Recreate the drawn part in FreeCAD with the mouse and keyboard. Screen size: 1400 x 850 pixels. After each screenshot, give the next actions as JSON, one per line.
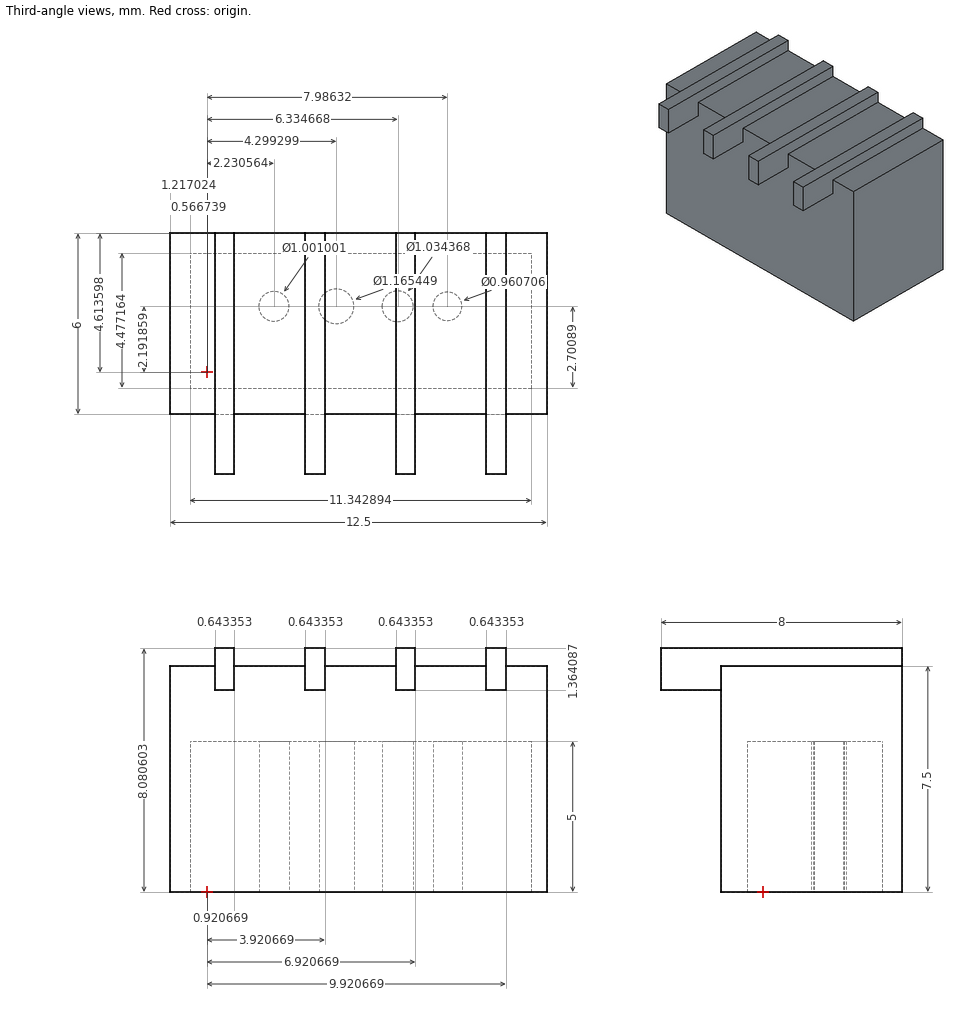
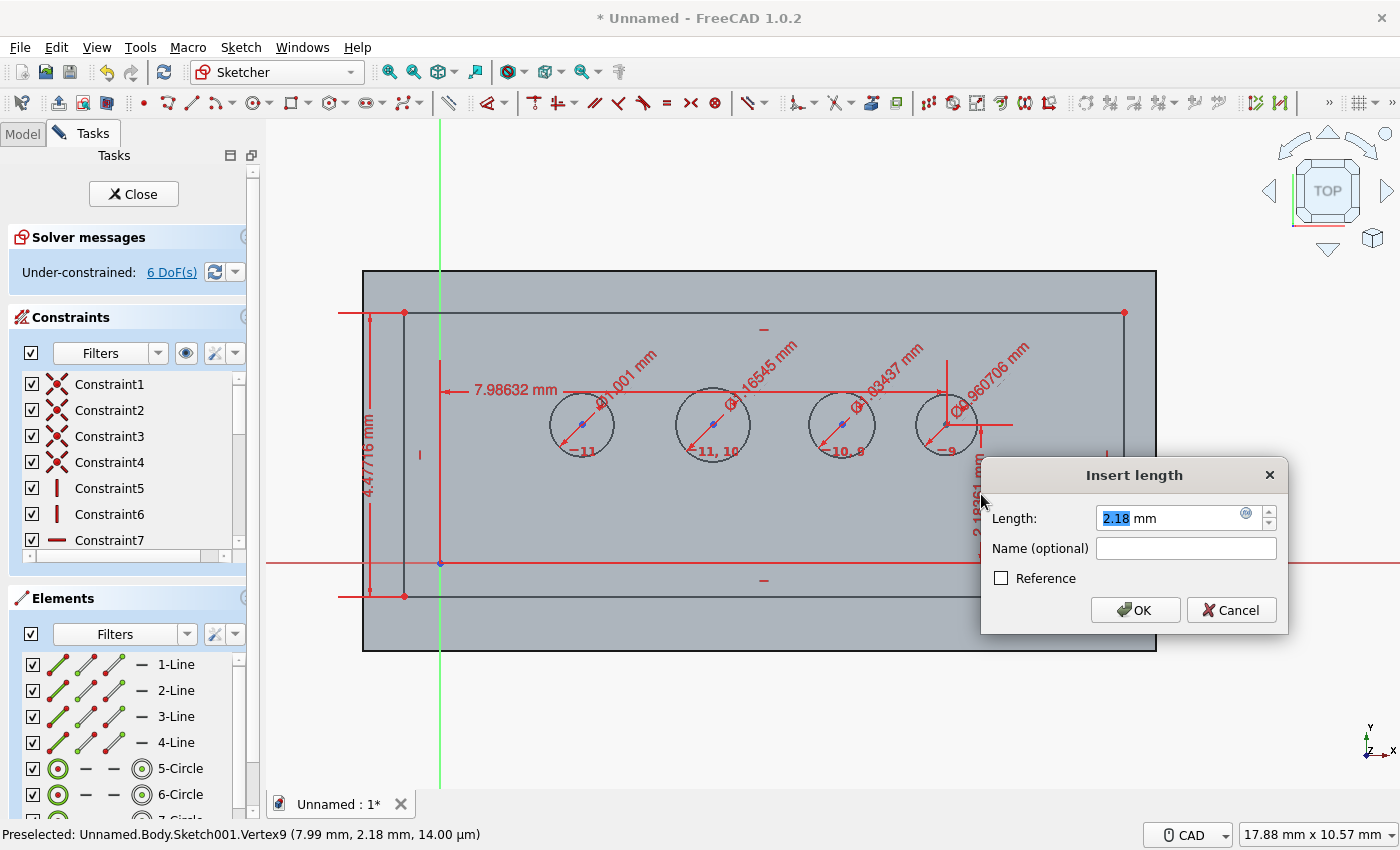
{"action": "type", "text": "2.191859"}
{"action": "key", "text": "Return"}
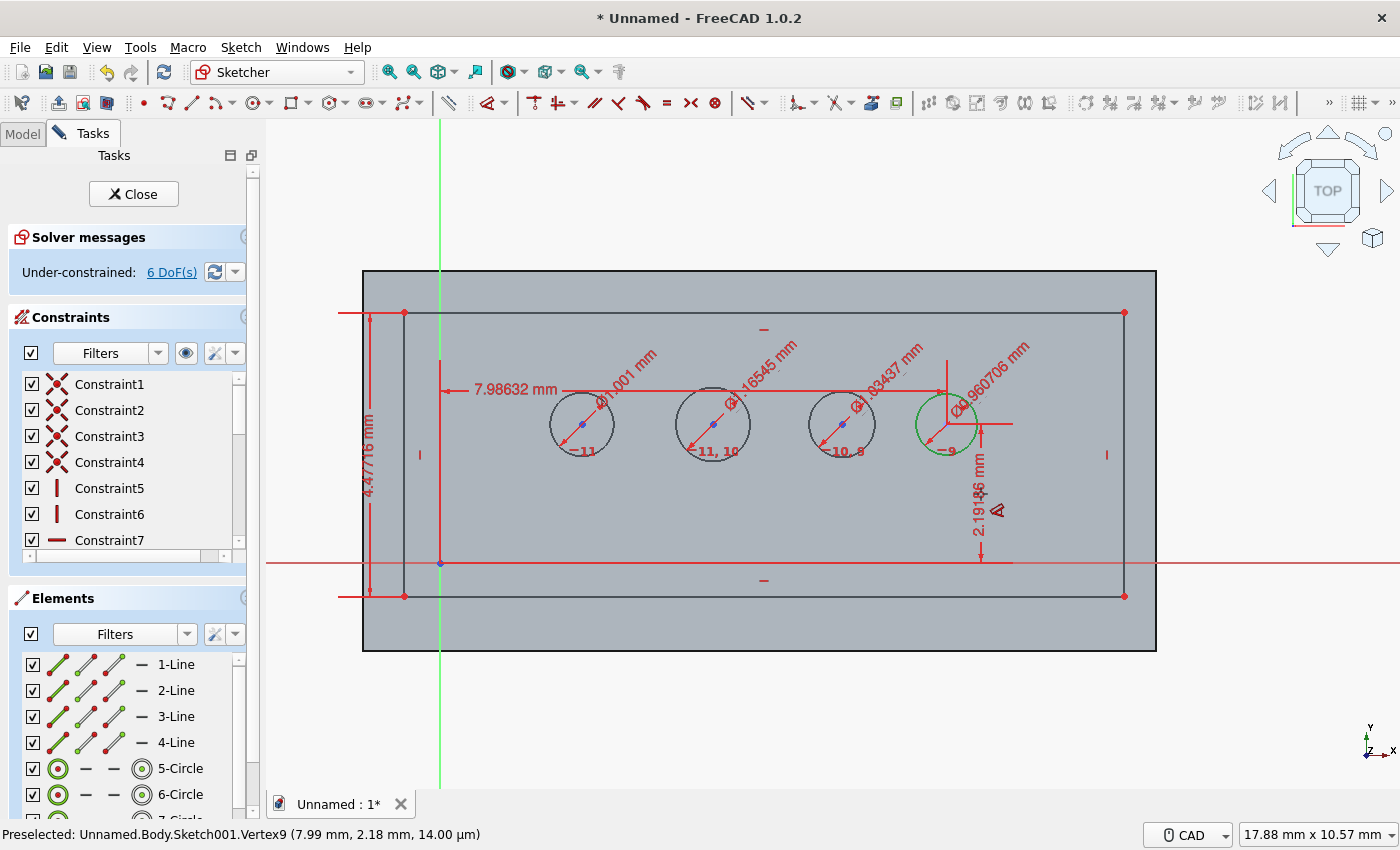
{"action": "left_click", "coordinate": [842, 424]}
{"action": "left_click", "coordinate": [641, 621]}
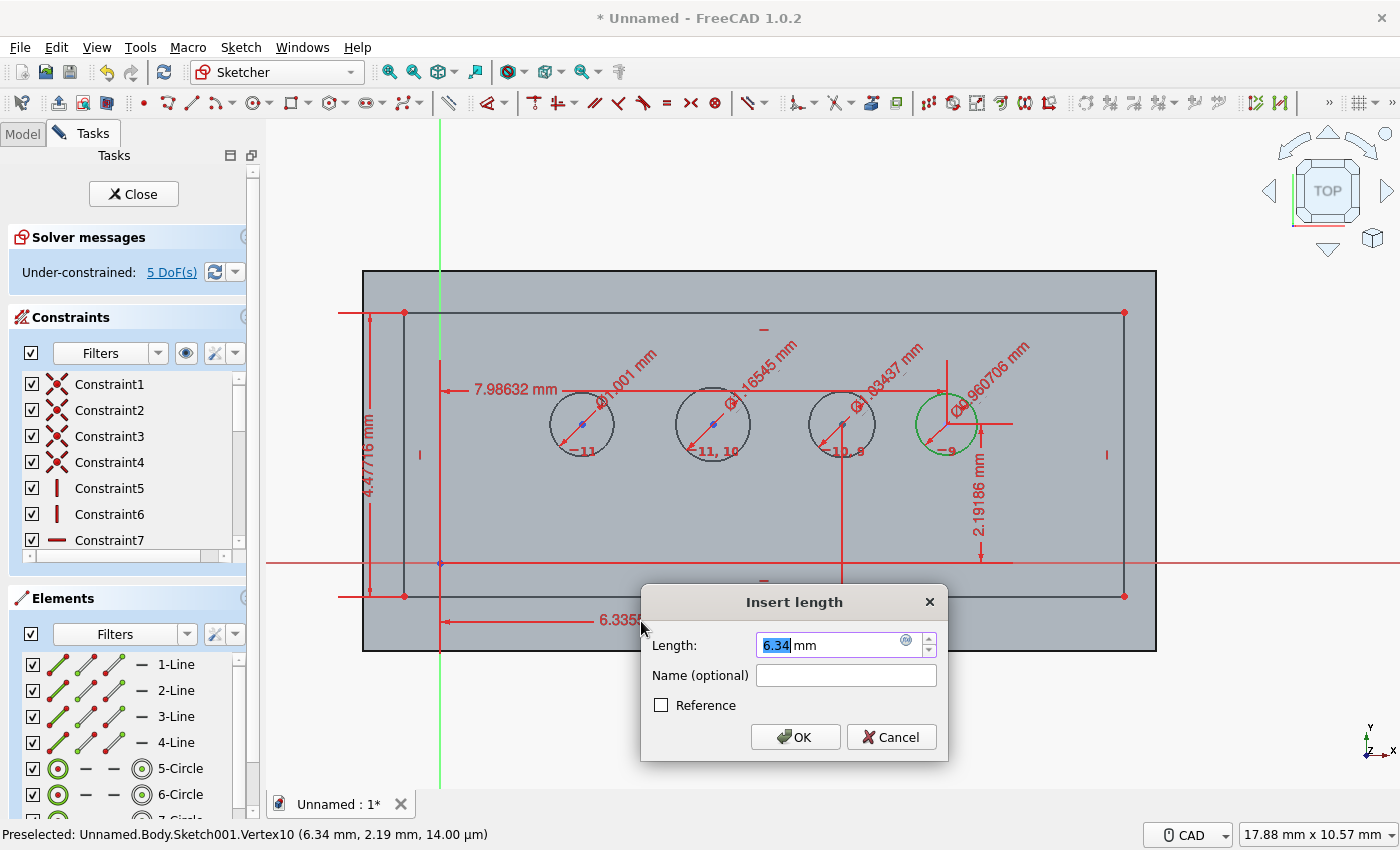
{"action": "type", "text": "6.334668"}
{"action": "key", "text": "Return"}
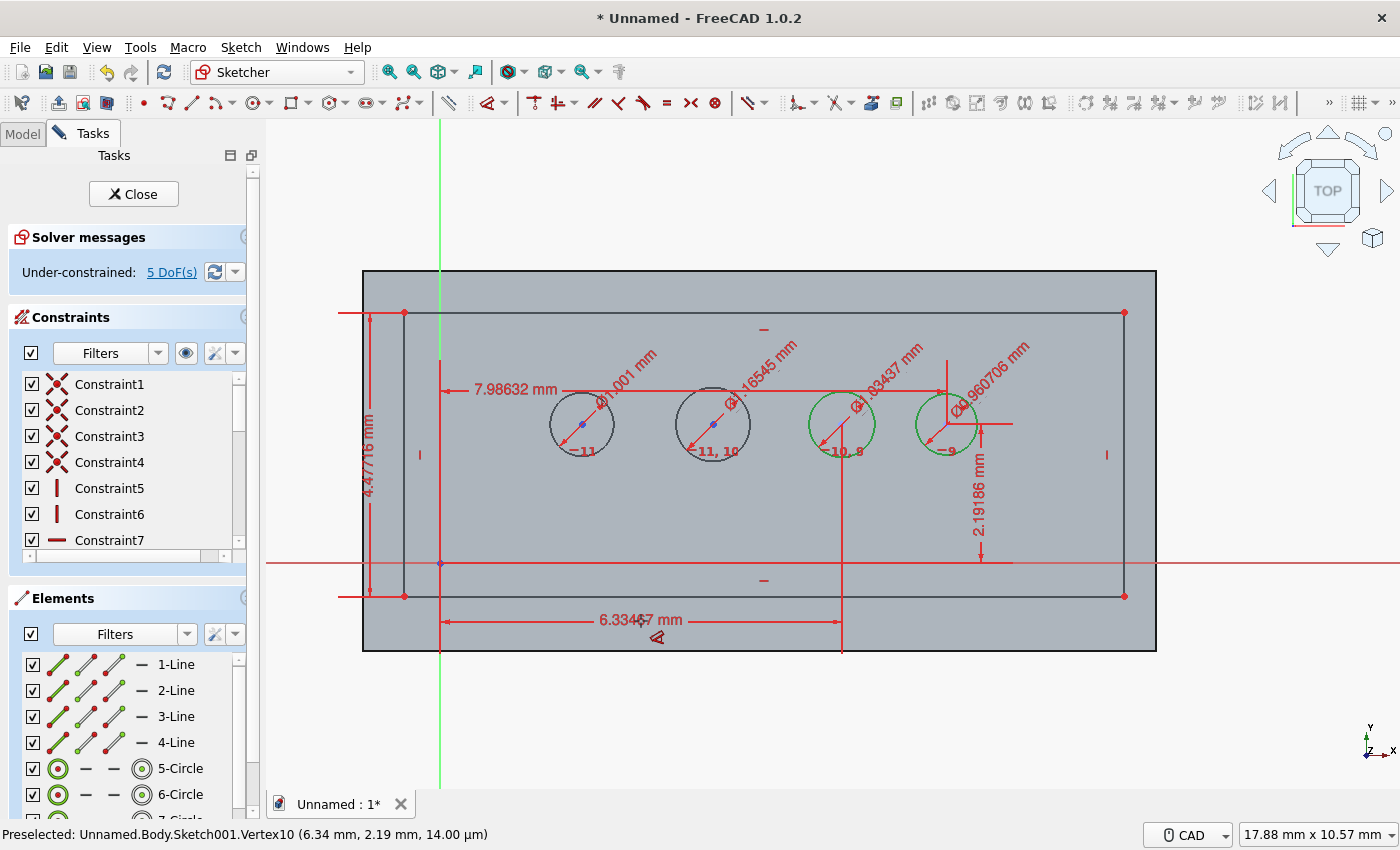
{"action": "left_click", "coordinate": [713, 424]}
{"action": "left_click", "coordinate": [514, 621]}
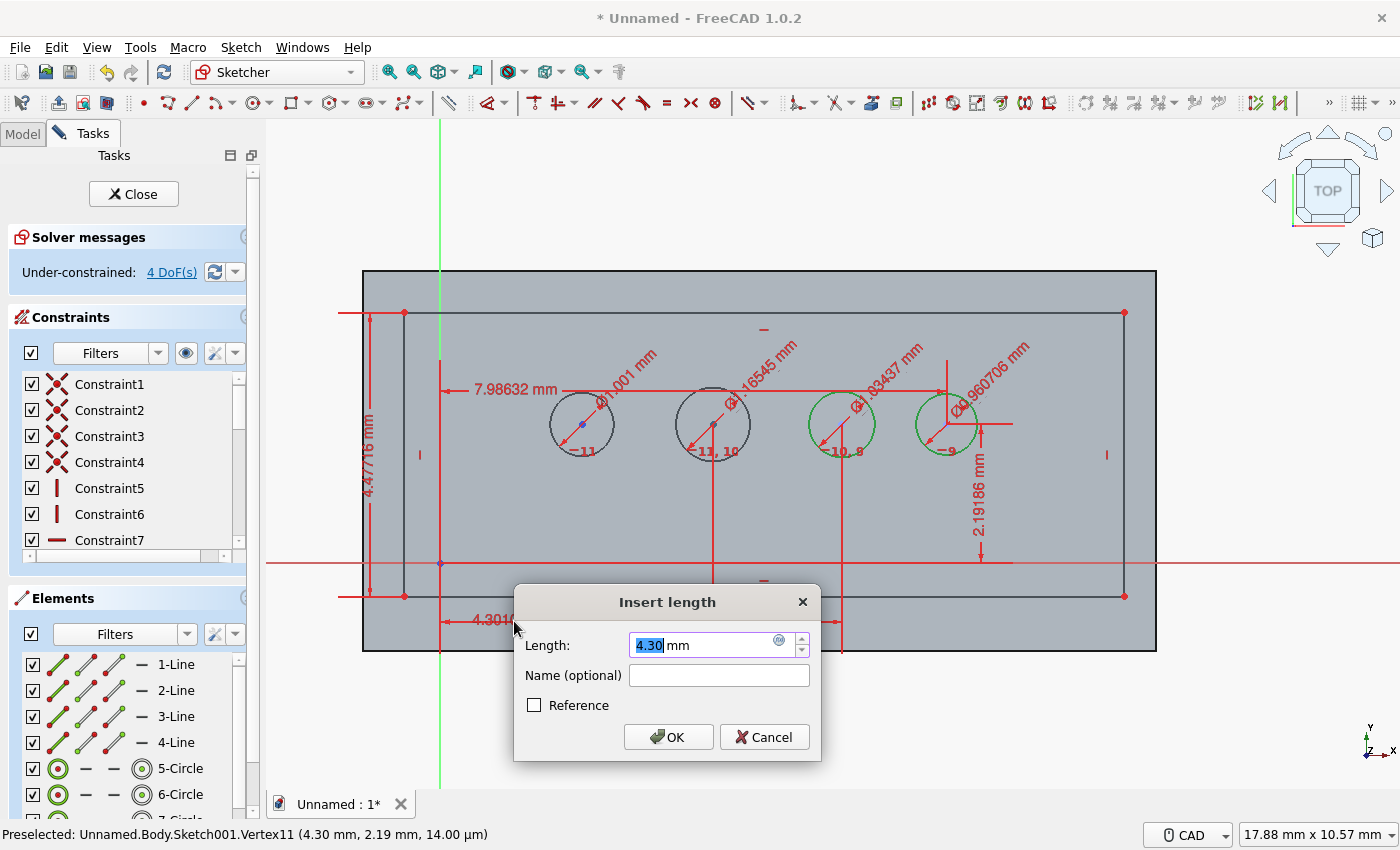
{"action": "type", "text": "4.299299"}
{"action": "key", "text": "Return"}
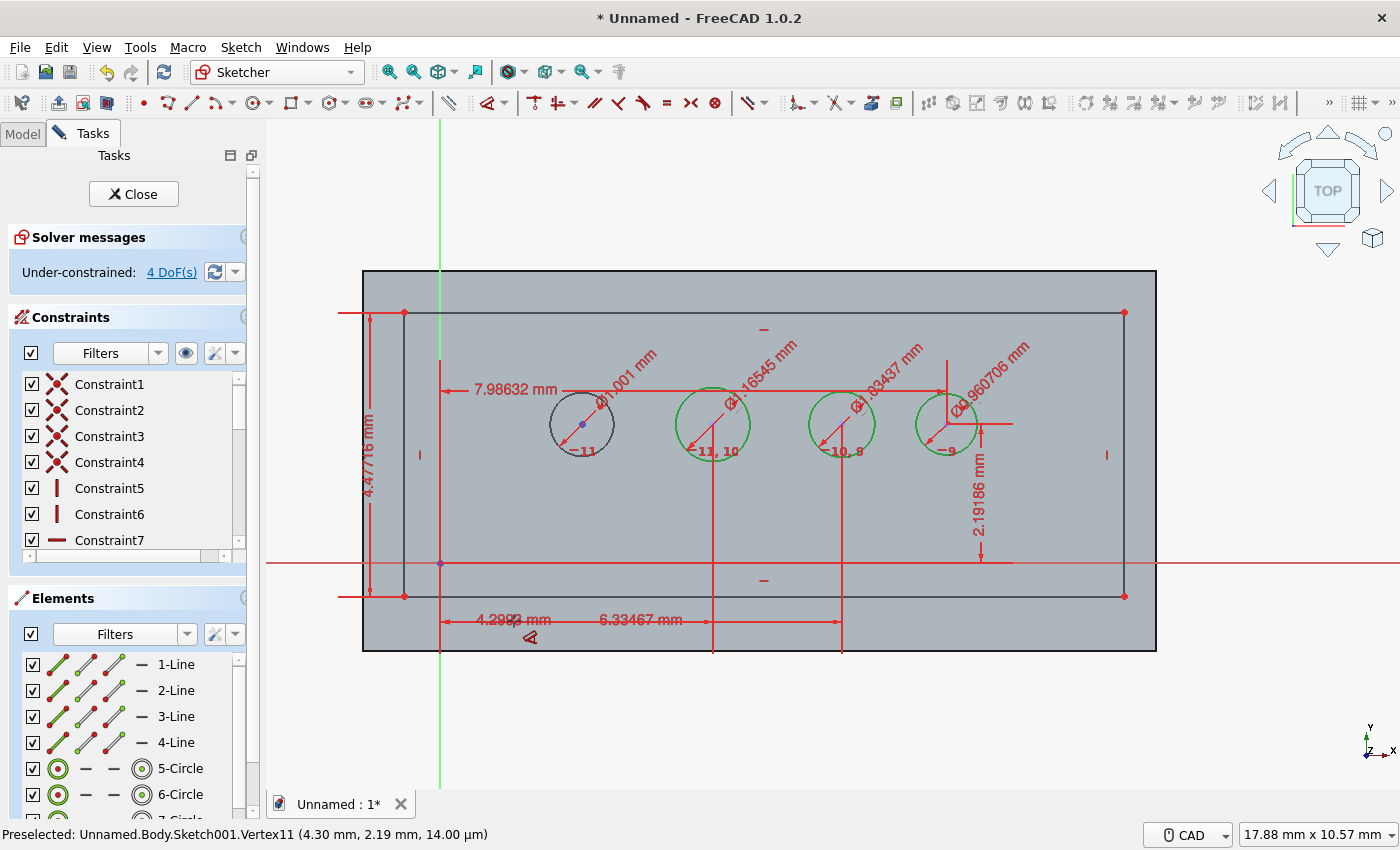
{"action": "left_click", "coordinate": [582, 424]}
{"action": "left_click", "coordinate": [511, 366]}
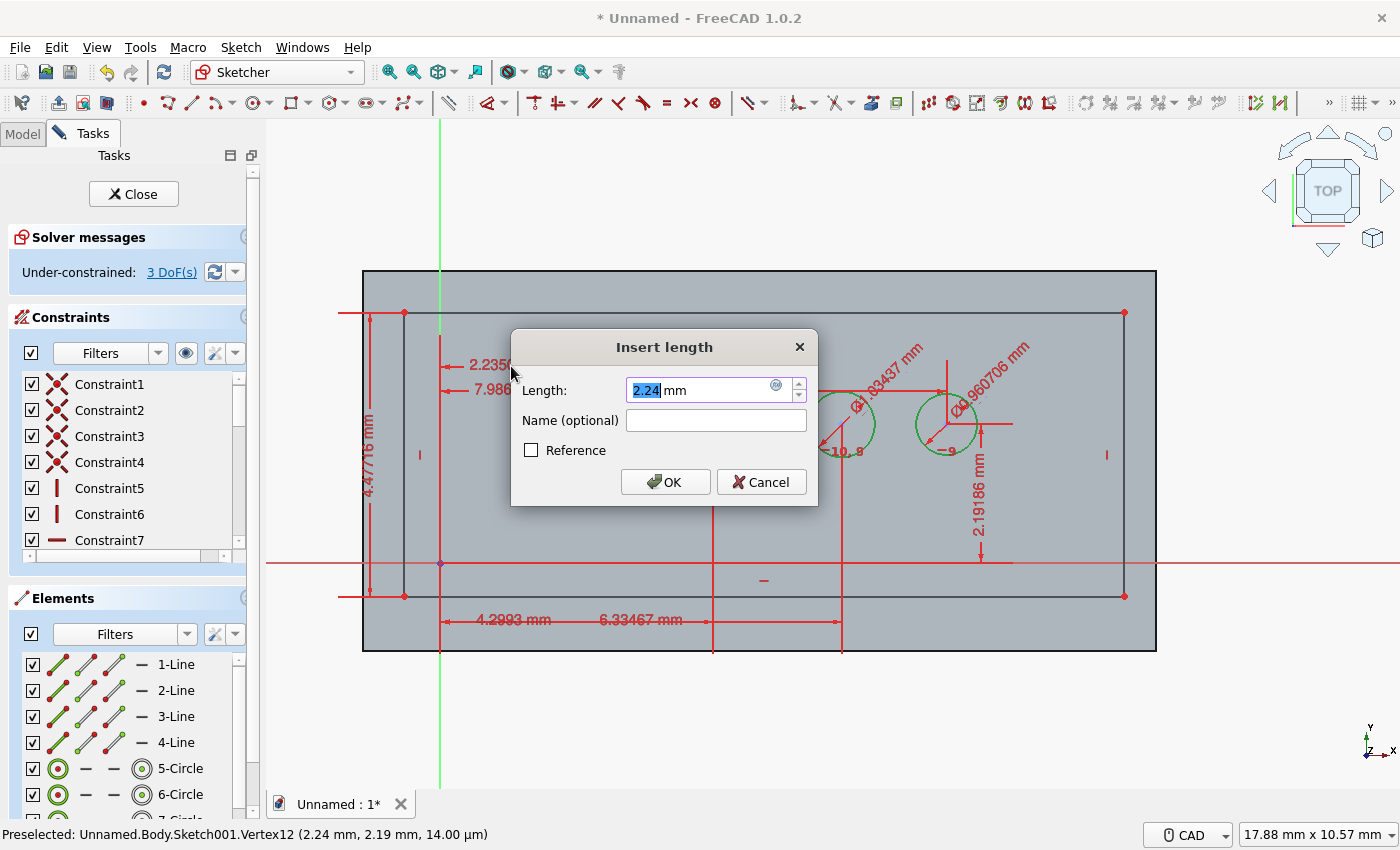
{"action": "type", "text": "2.230564"}
{"action": "key", "text": "Return"}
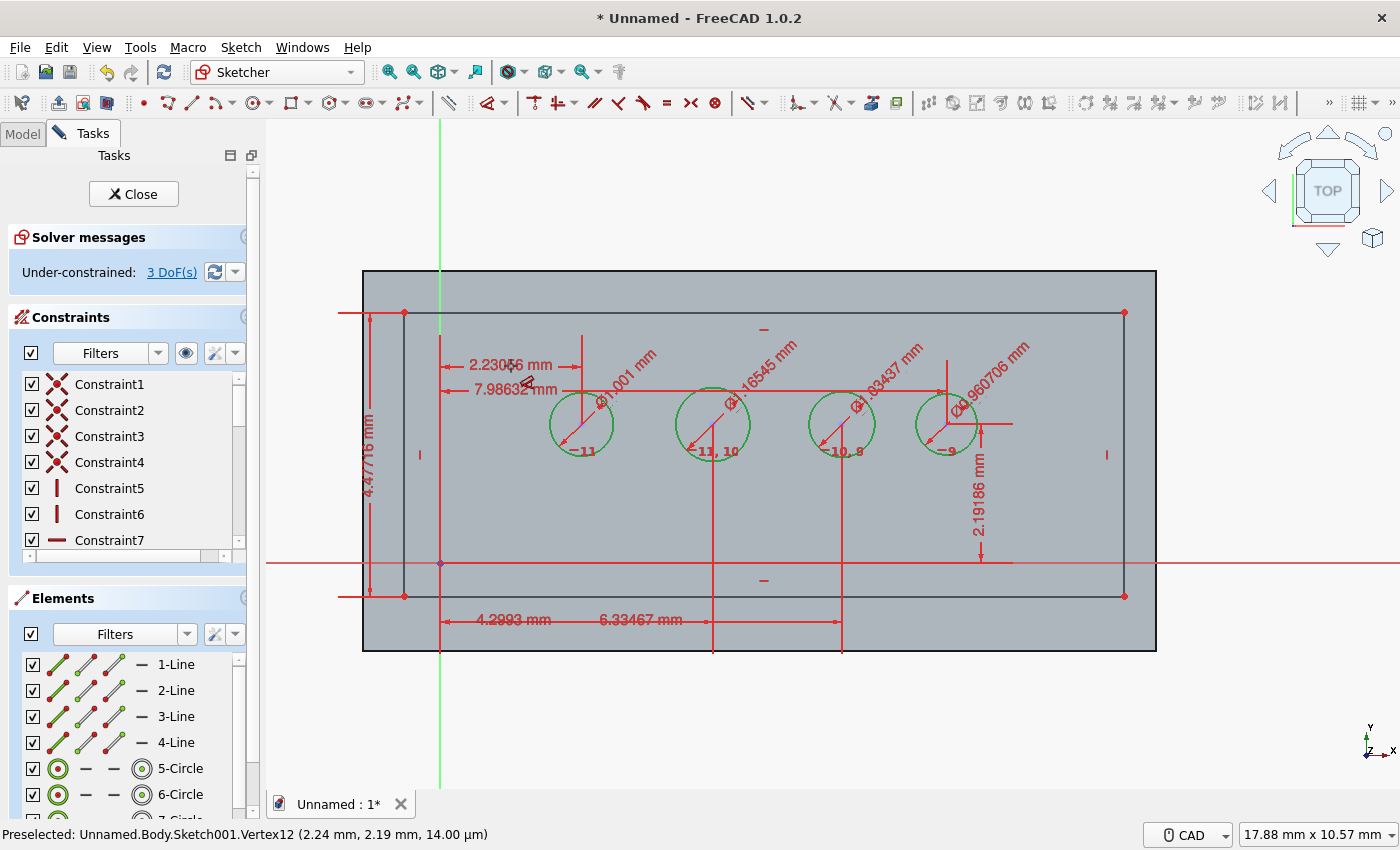
{"action": "left_click", "coordinate": [1124, 597]}